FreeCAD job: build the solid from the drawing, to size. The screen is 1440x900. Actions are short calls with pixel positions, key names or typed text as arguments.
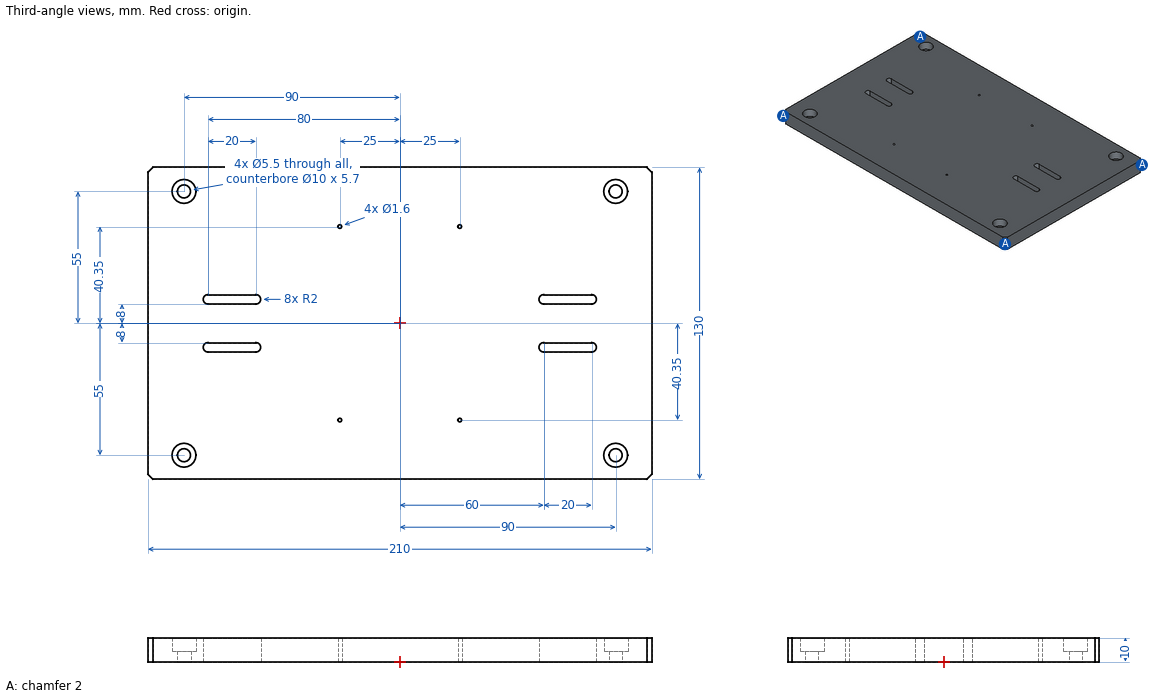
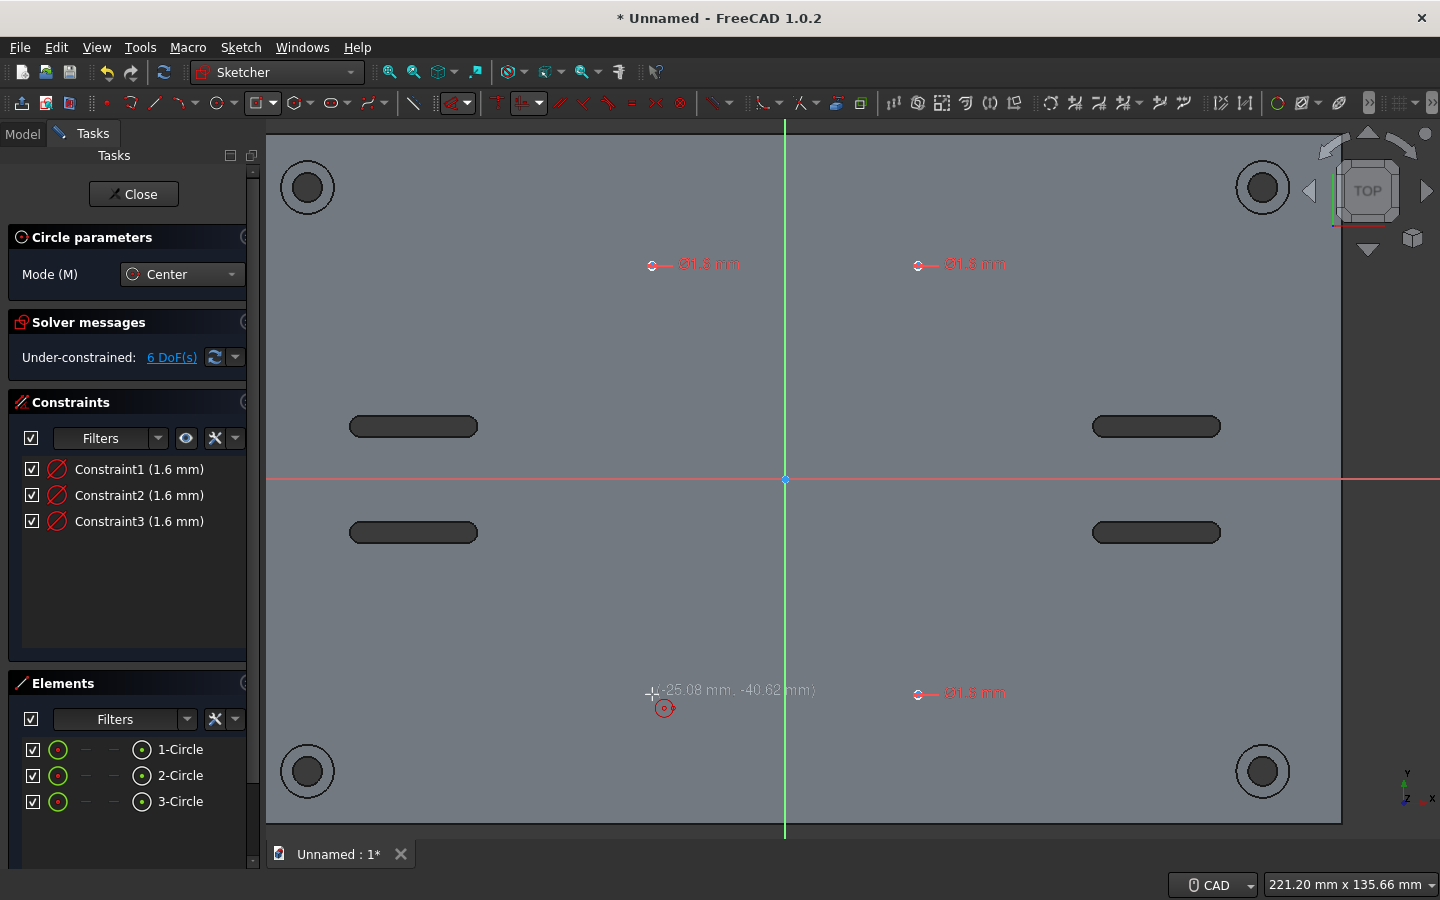
click(652, 694)
move(655, 691)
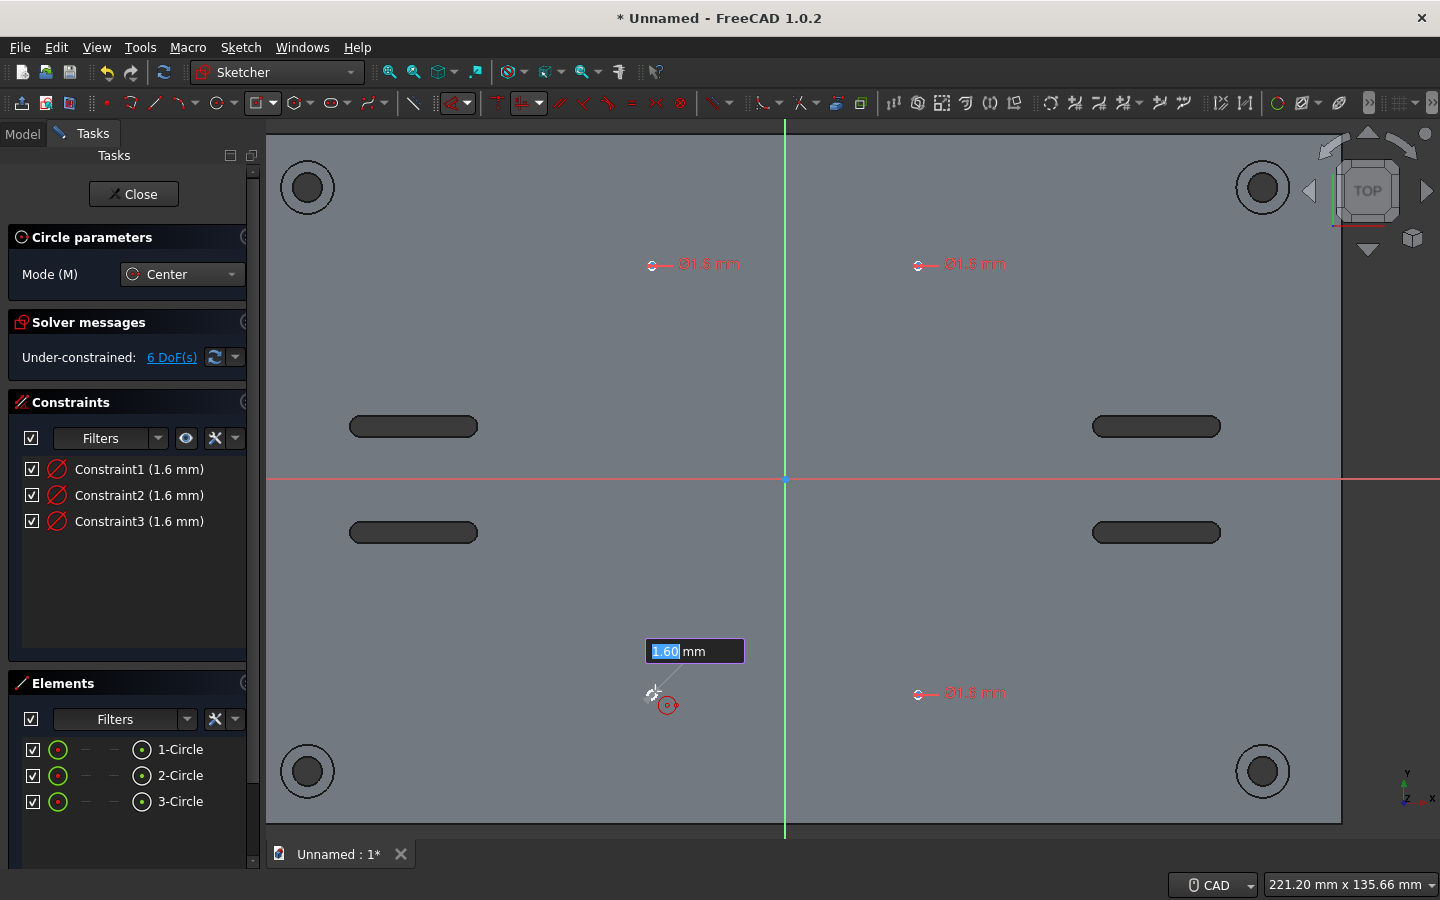
text(1.6)
key(Return)
key(Escape)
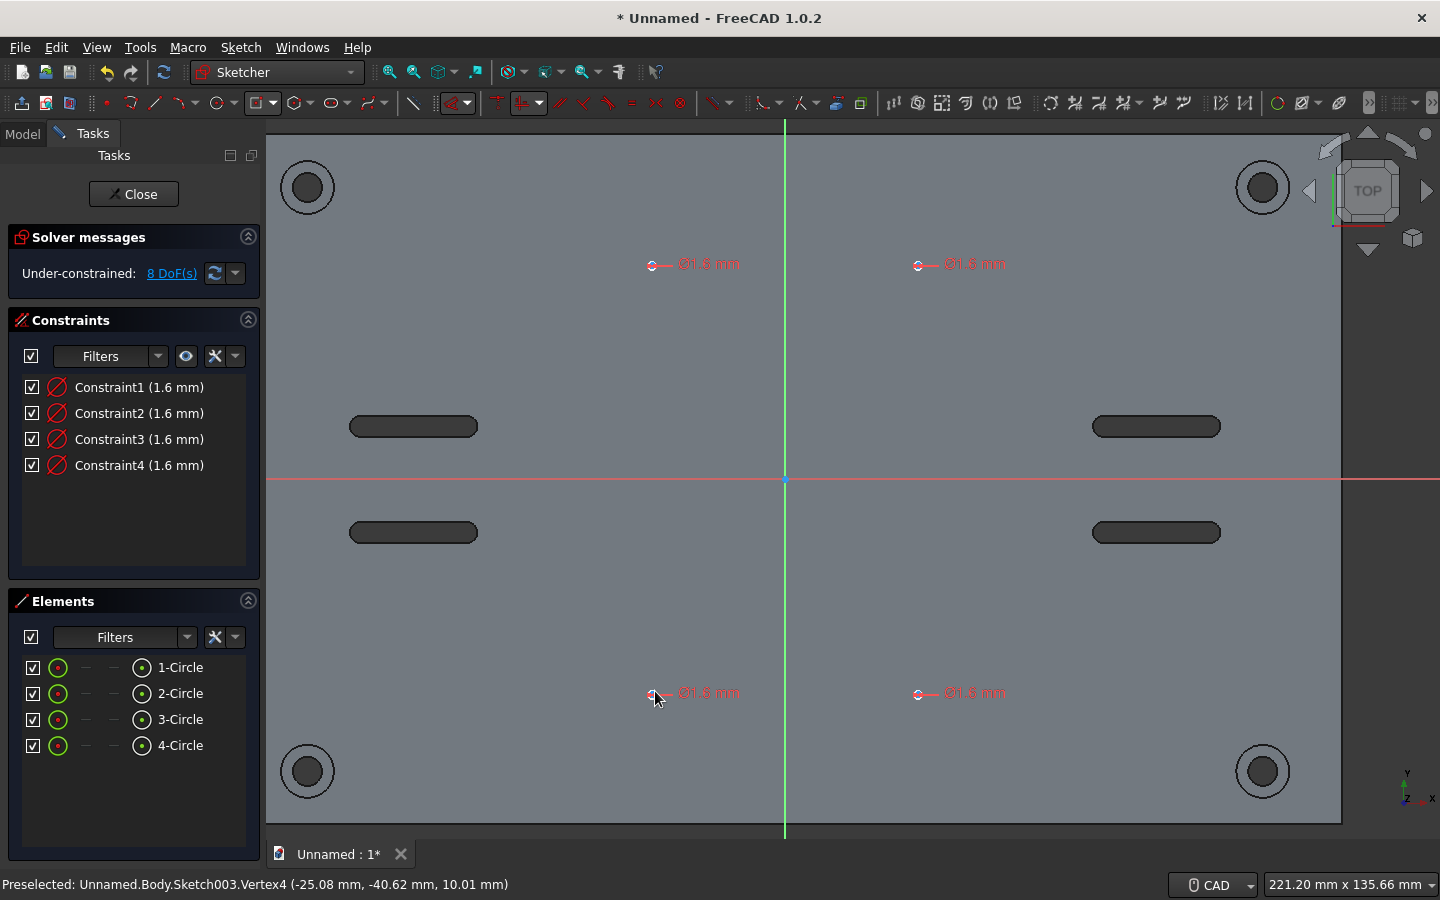
click(652, 266)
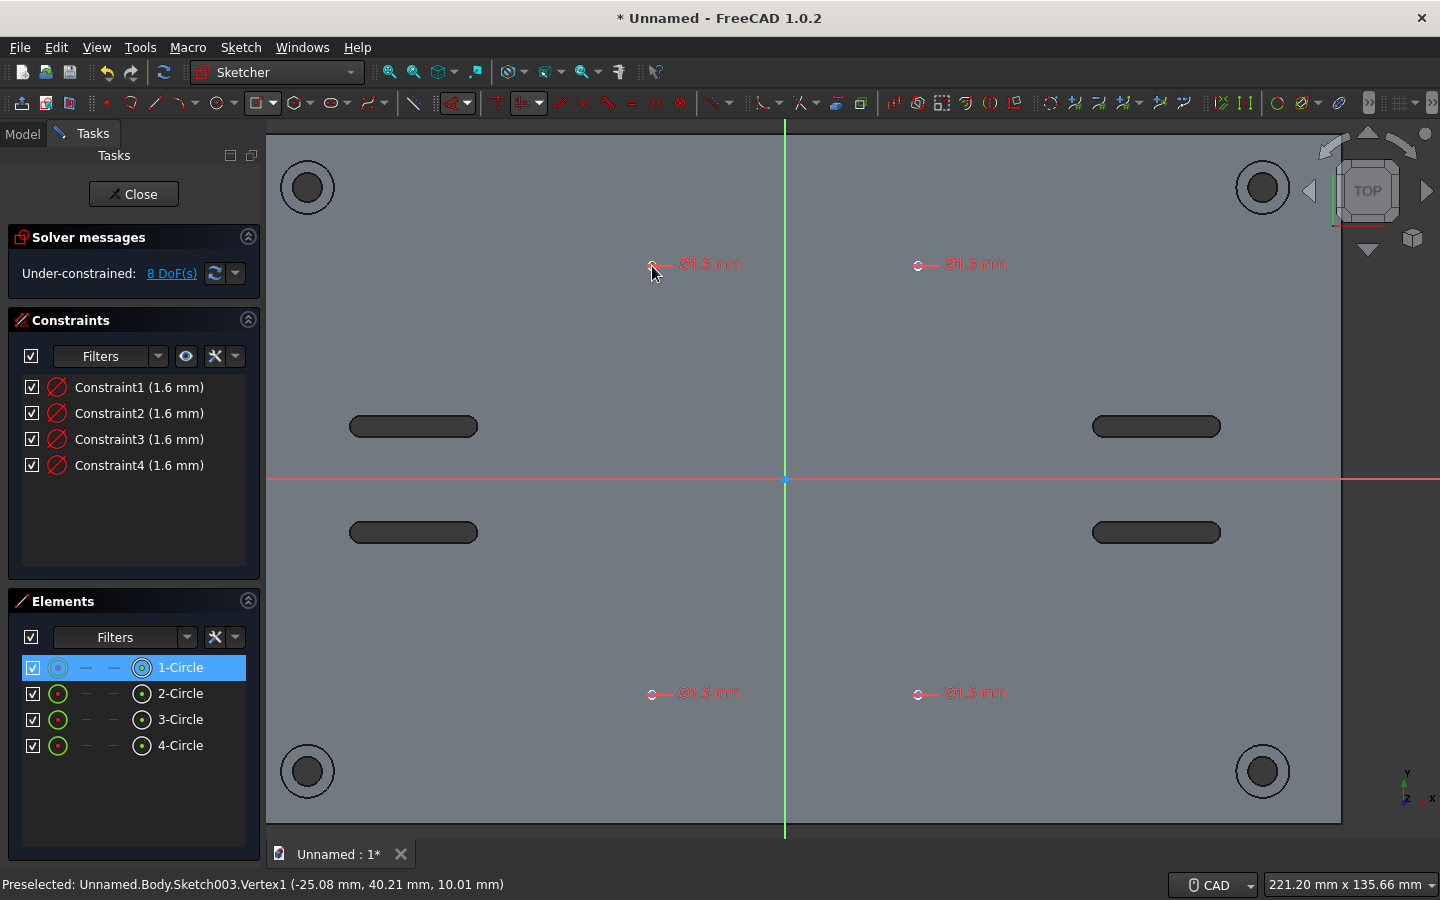
click(918, 266)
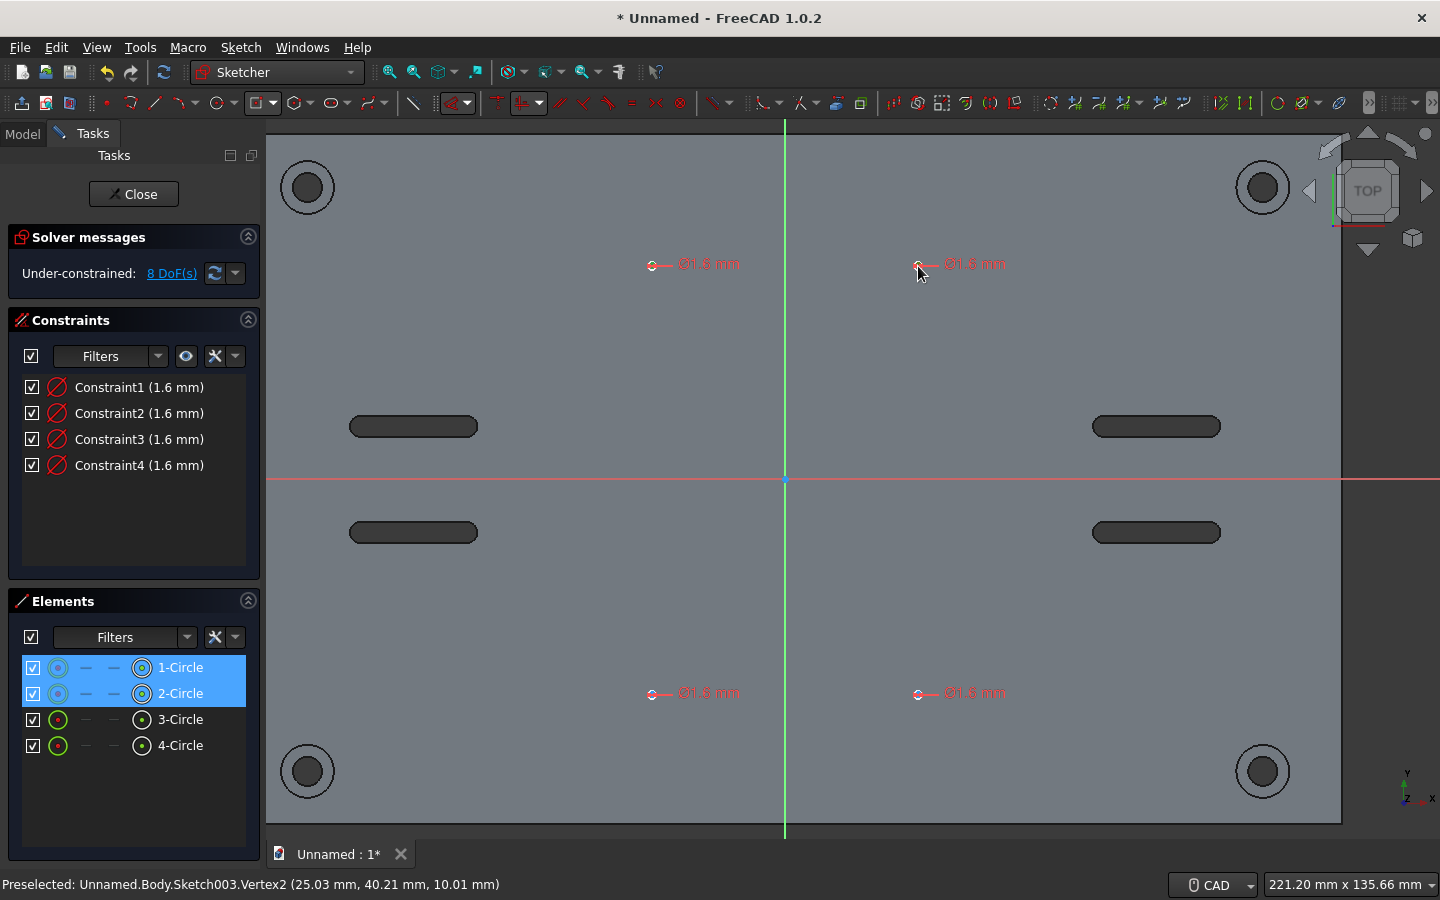
key(h)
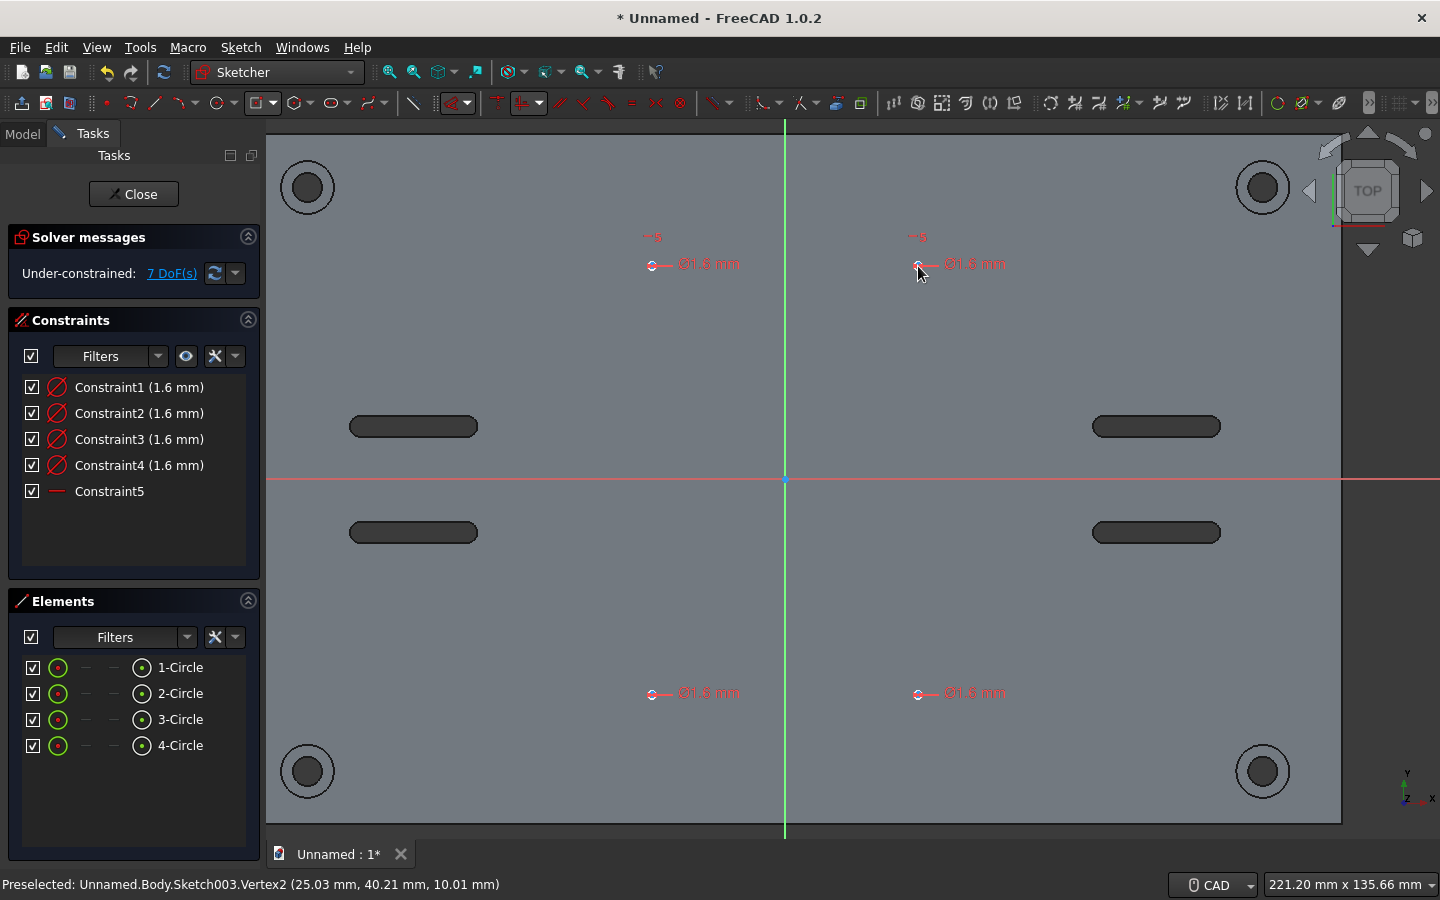
click(918, 266)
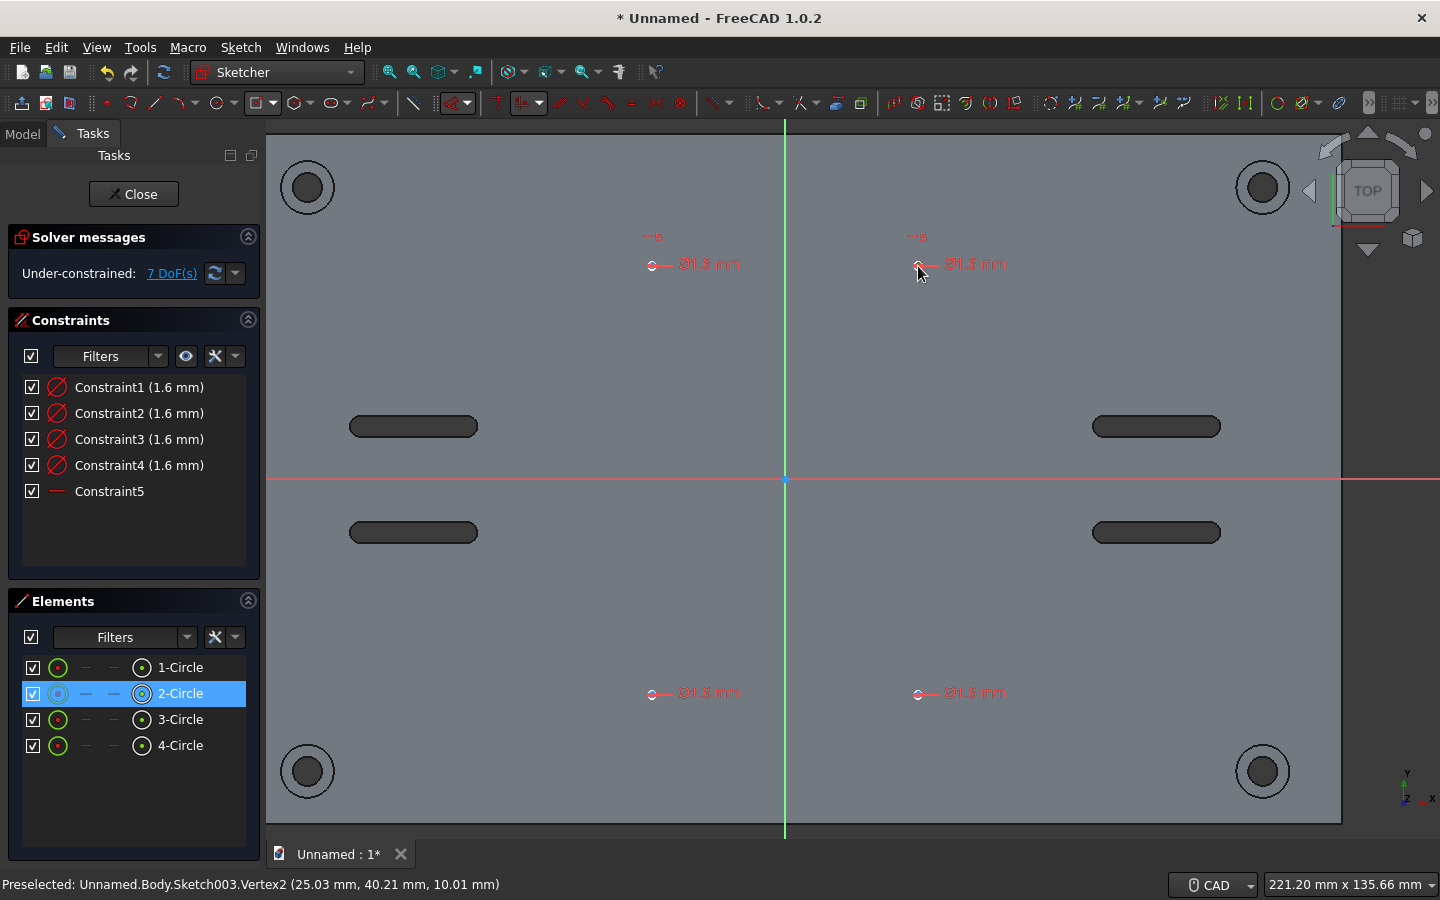
click(918, 695)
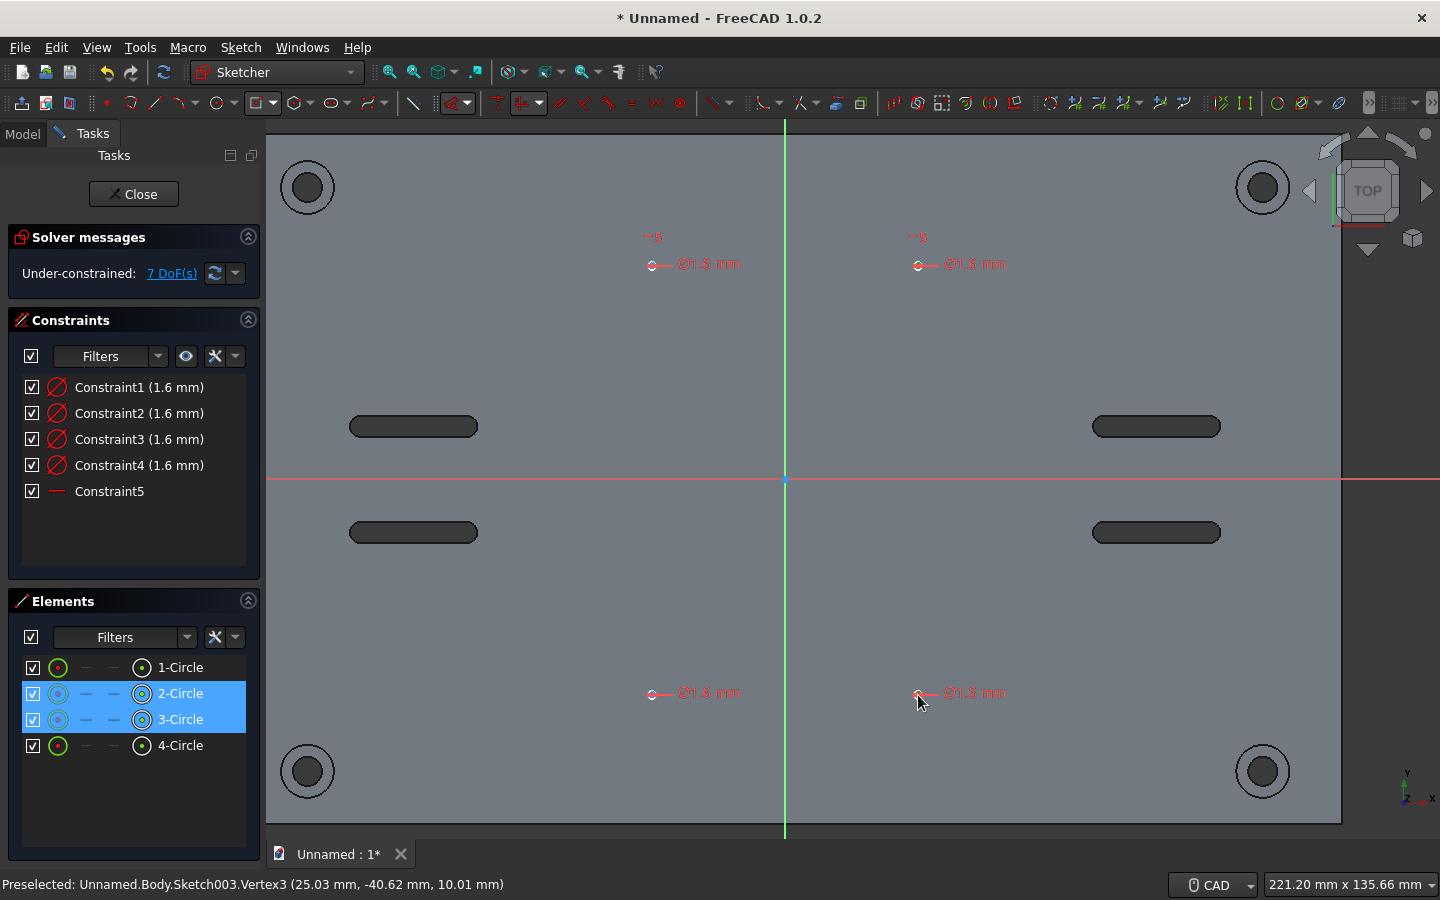
click(542, 104)